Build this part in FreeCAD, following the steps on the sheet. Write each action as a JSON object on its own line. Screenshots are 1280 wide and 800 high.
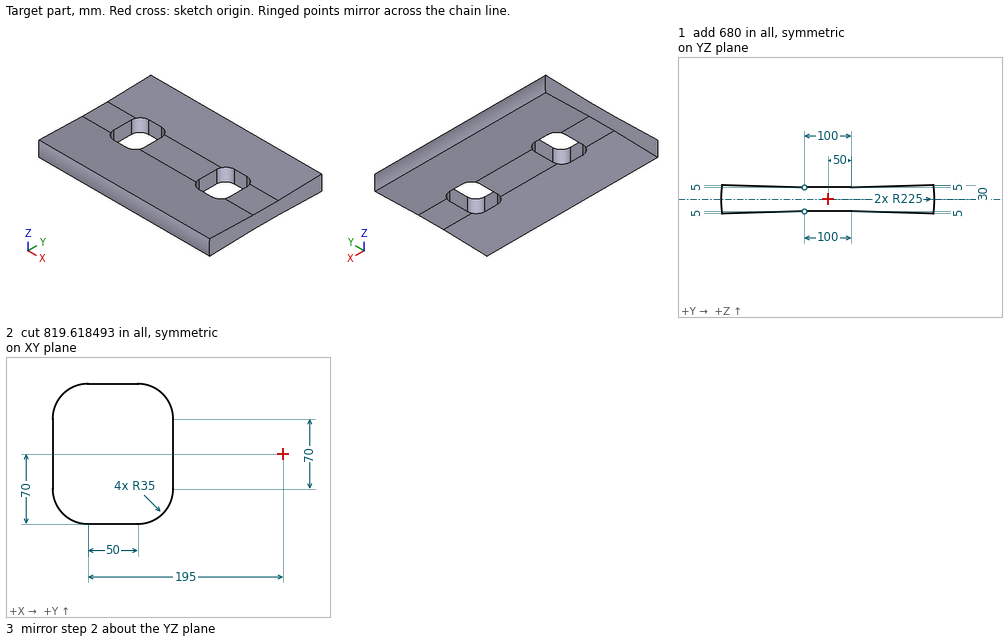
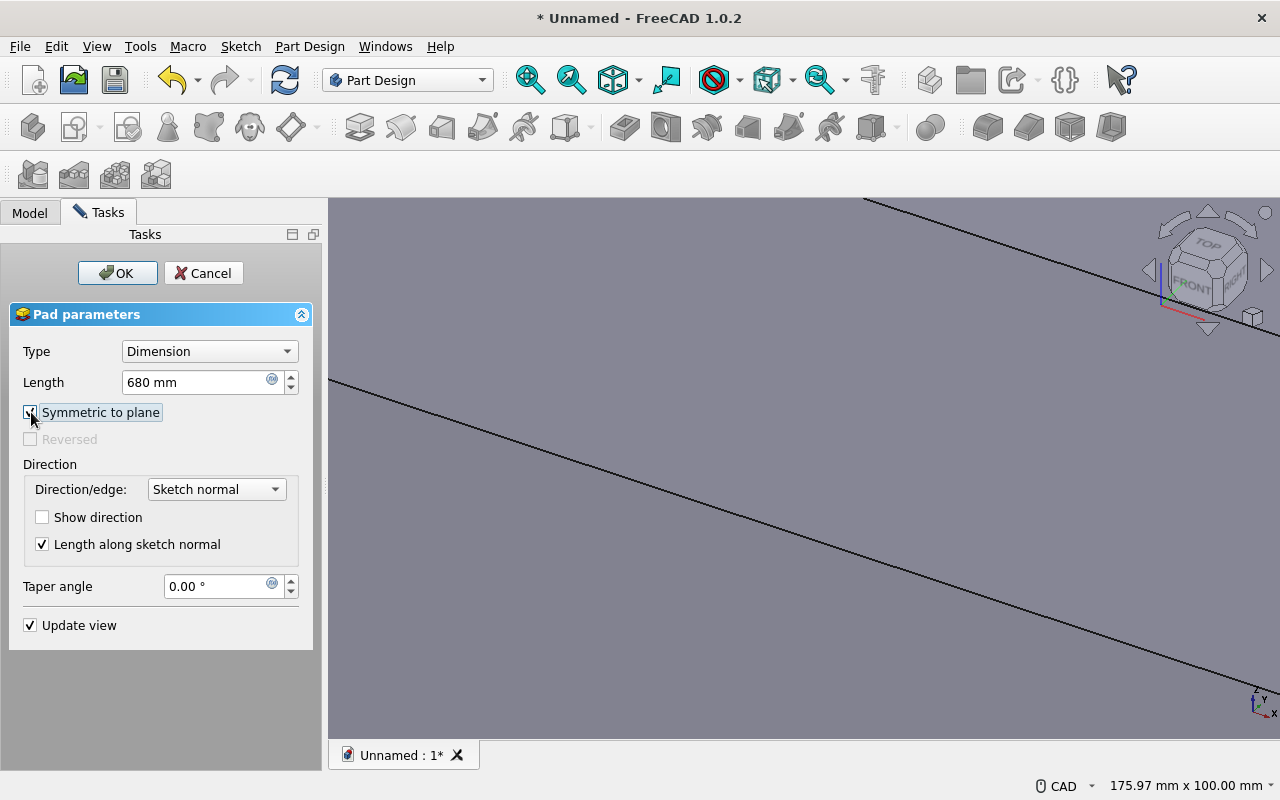
{"action": "left_click", "coordinate": [118, 273]}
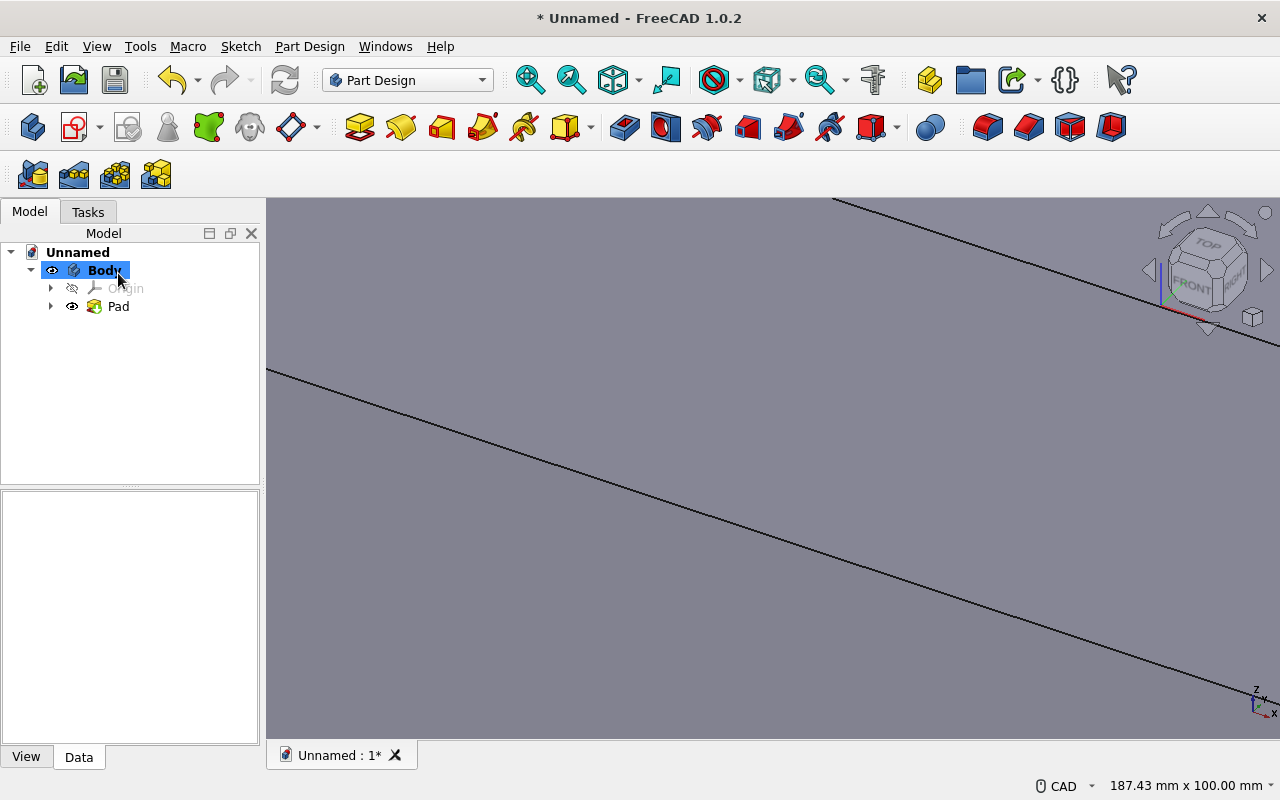
{"action": "key", "text": "v f"}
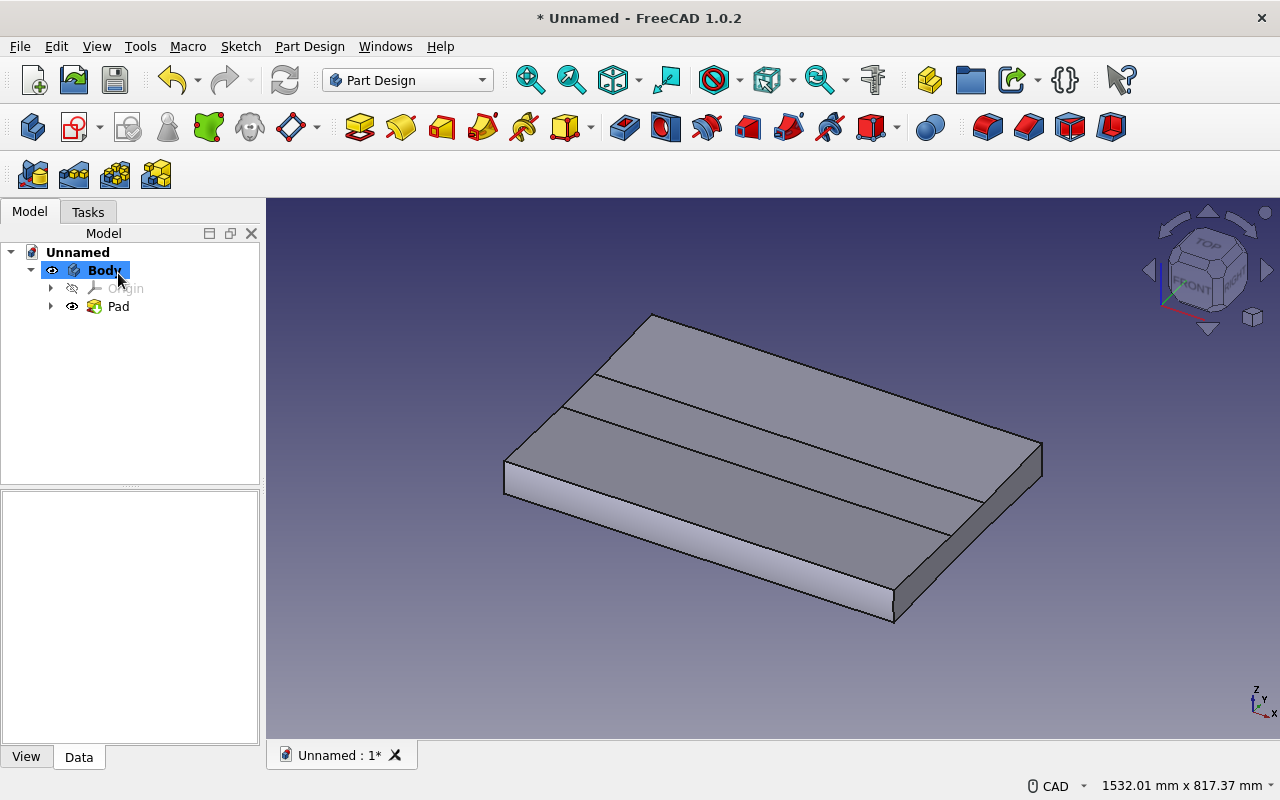
{"action": "left_click", "coordinate": [74, 128]}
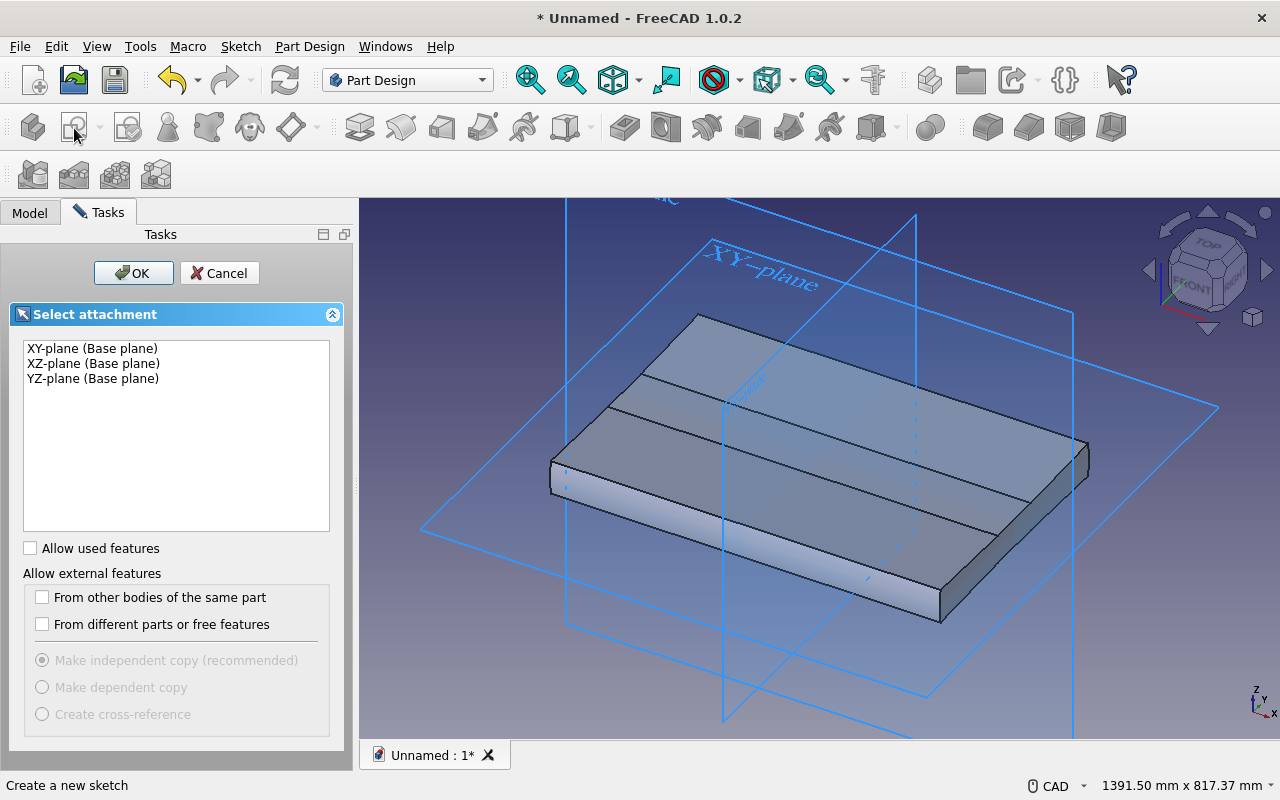
{"action": "left_click", "coordinate": [84, 348]}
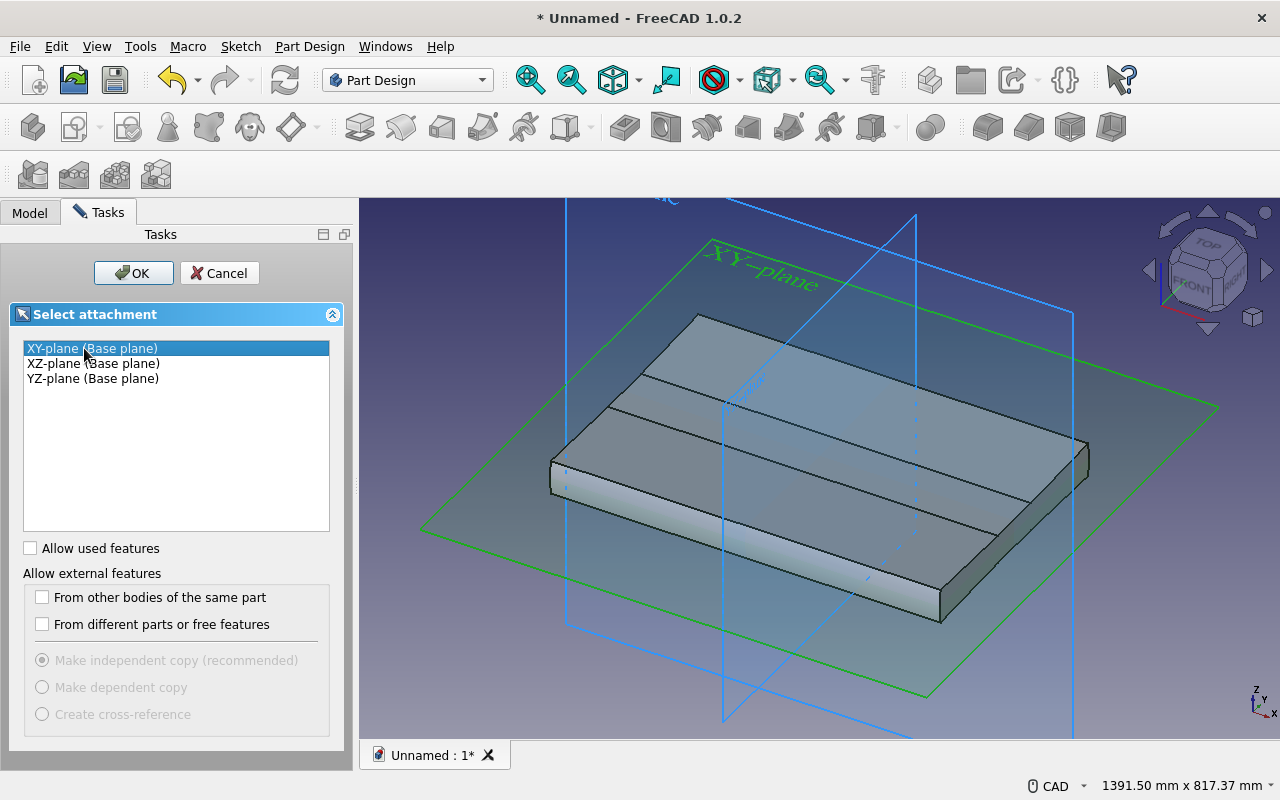
{"action": "left_click", "coordinate": [134, 273]}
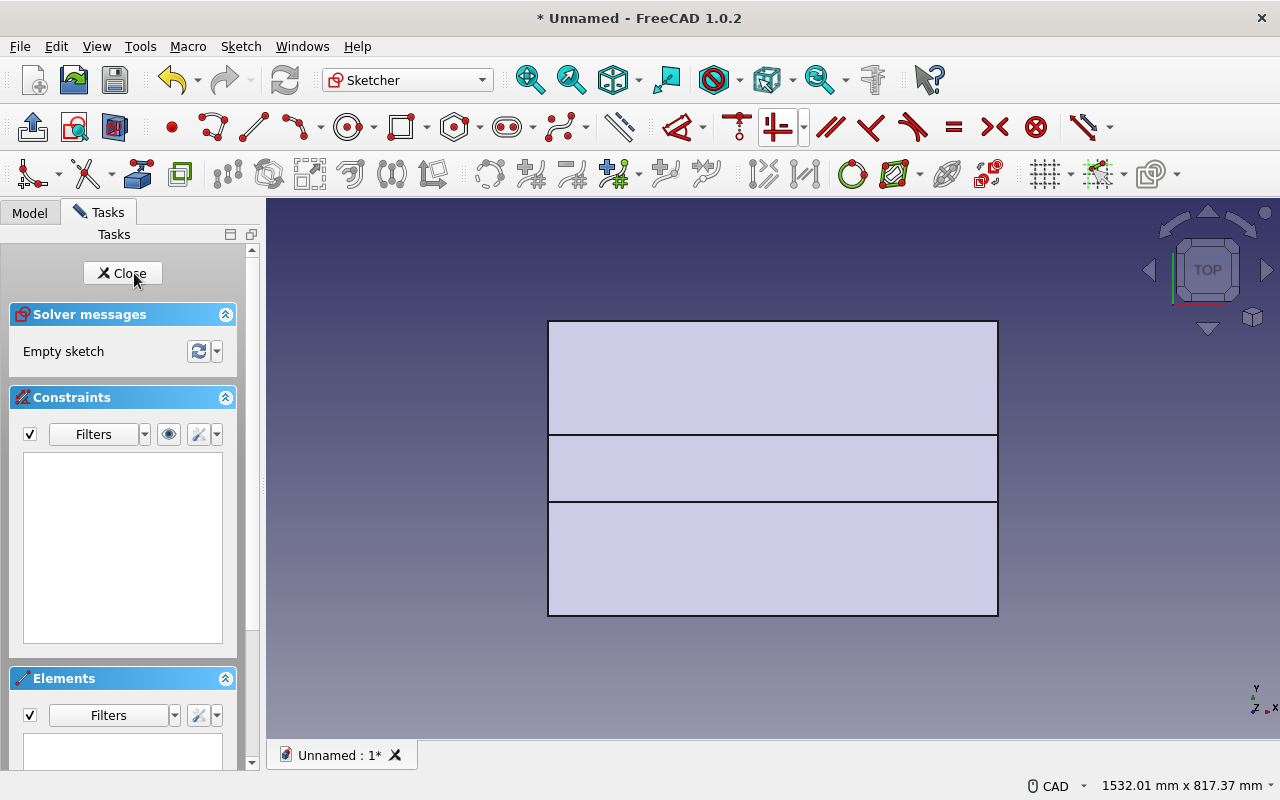
{"action": "left_click", "coordinate": [115, 128]}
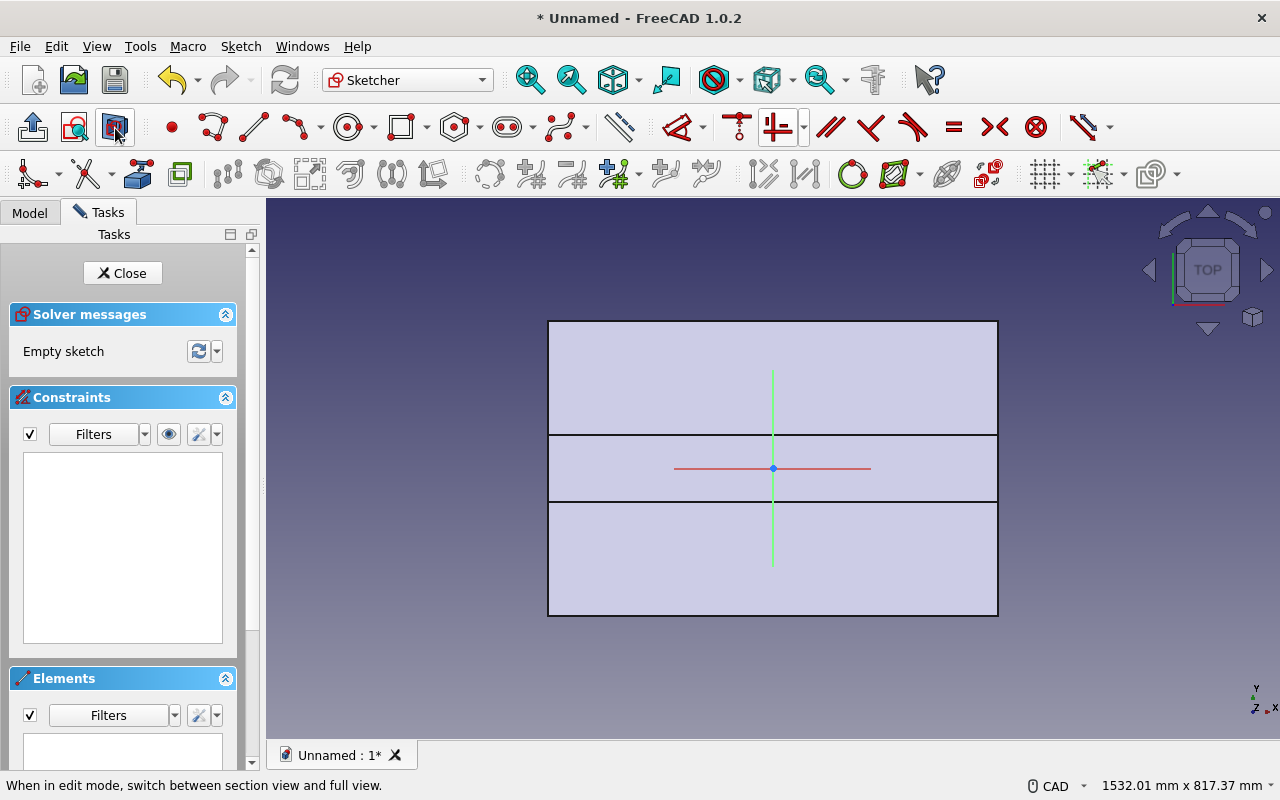
{"action": "scroll", "coordinate": [694, 468], "scroll_direction": "up", "scroll_amount": 7}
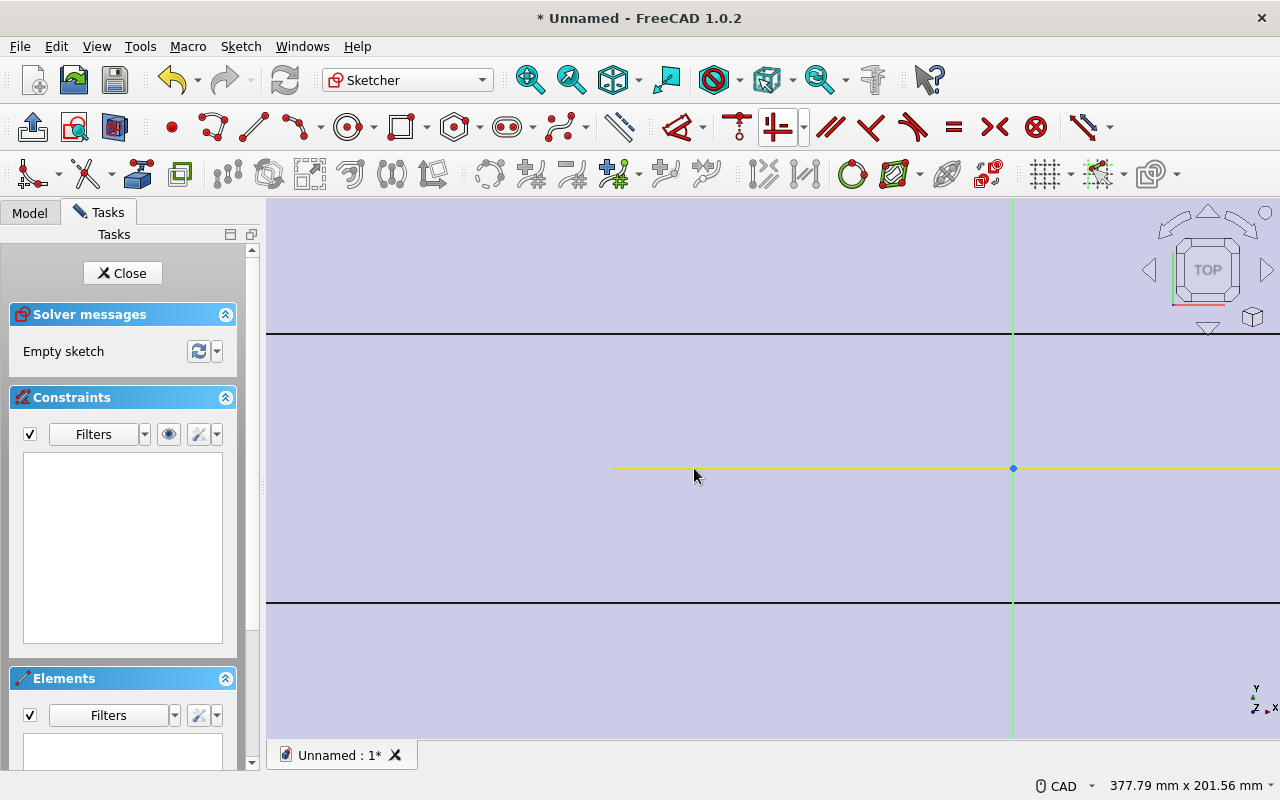
{"action": "left_click", "coordinate": [254, 128]}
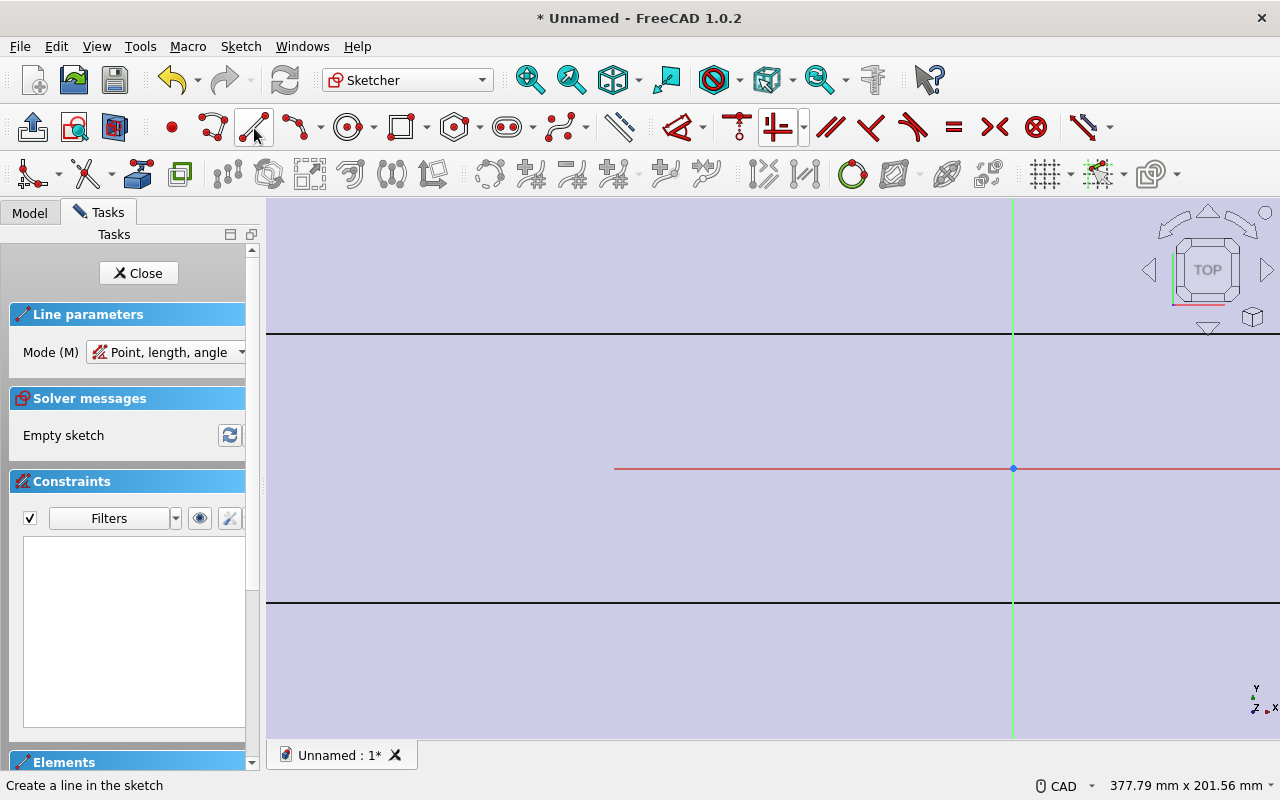
{"action": "left_click", "coordinate": [490, 656]}
{"action": "left_click", "coordinate": [624, 656]}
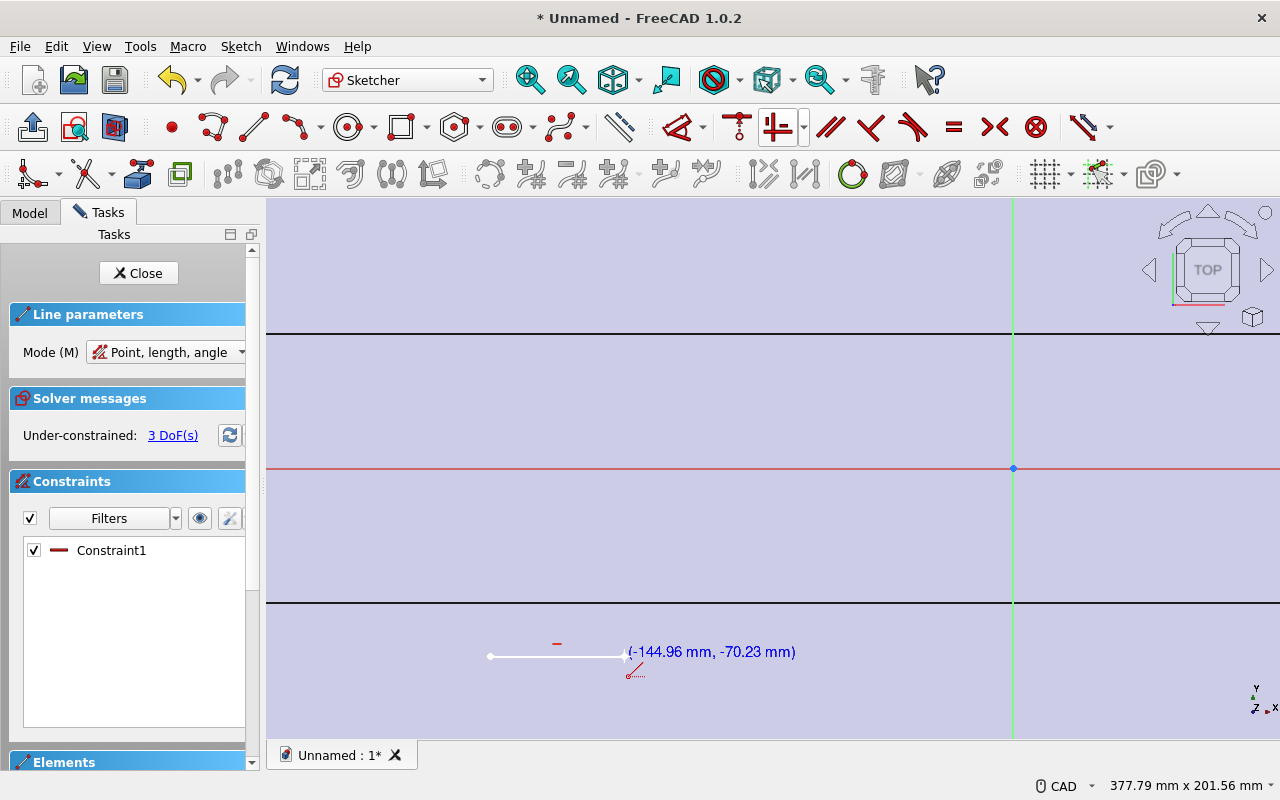
{"action": "left_click", "coordinate": [718, 562]}
{"action": "left_click", "coordinate": [718, 375]}